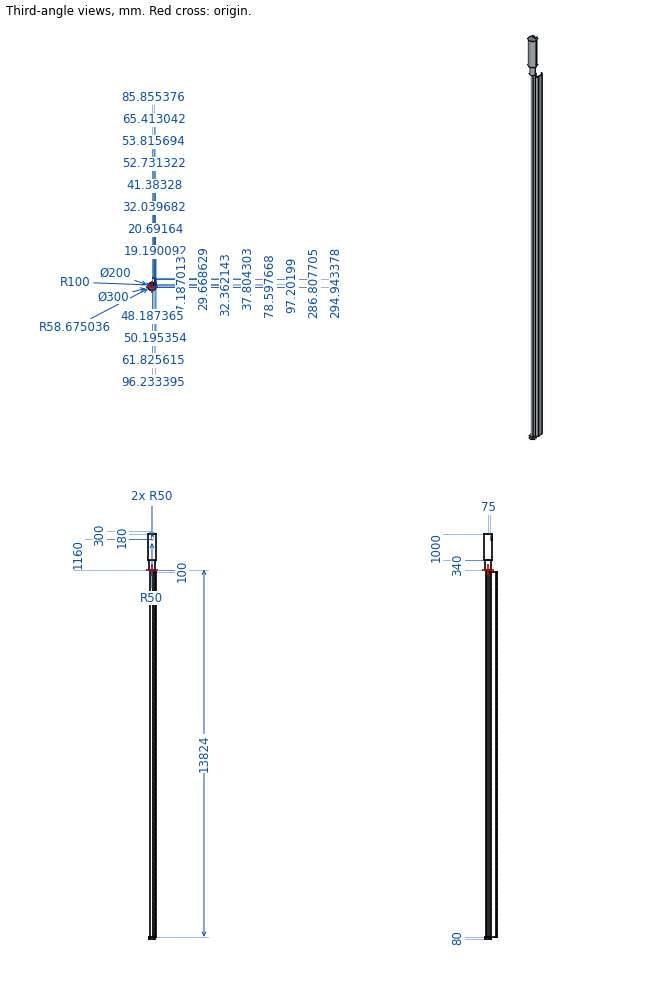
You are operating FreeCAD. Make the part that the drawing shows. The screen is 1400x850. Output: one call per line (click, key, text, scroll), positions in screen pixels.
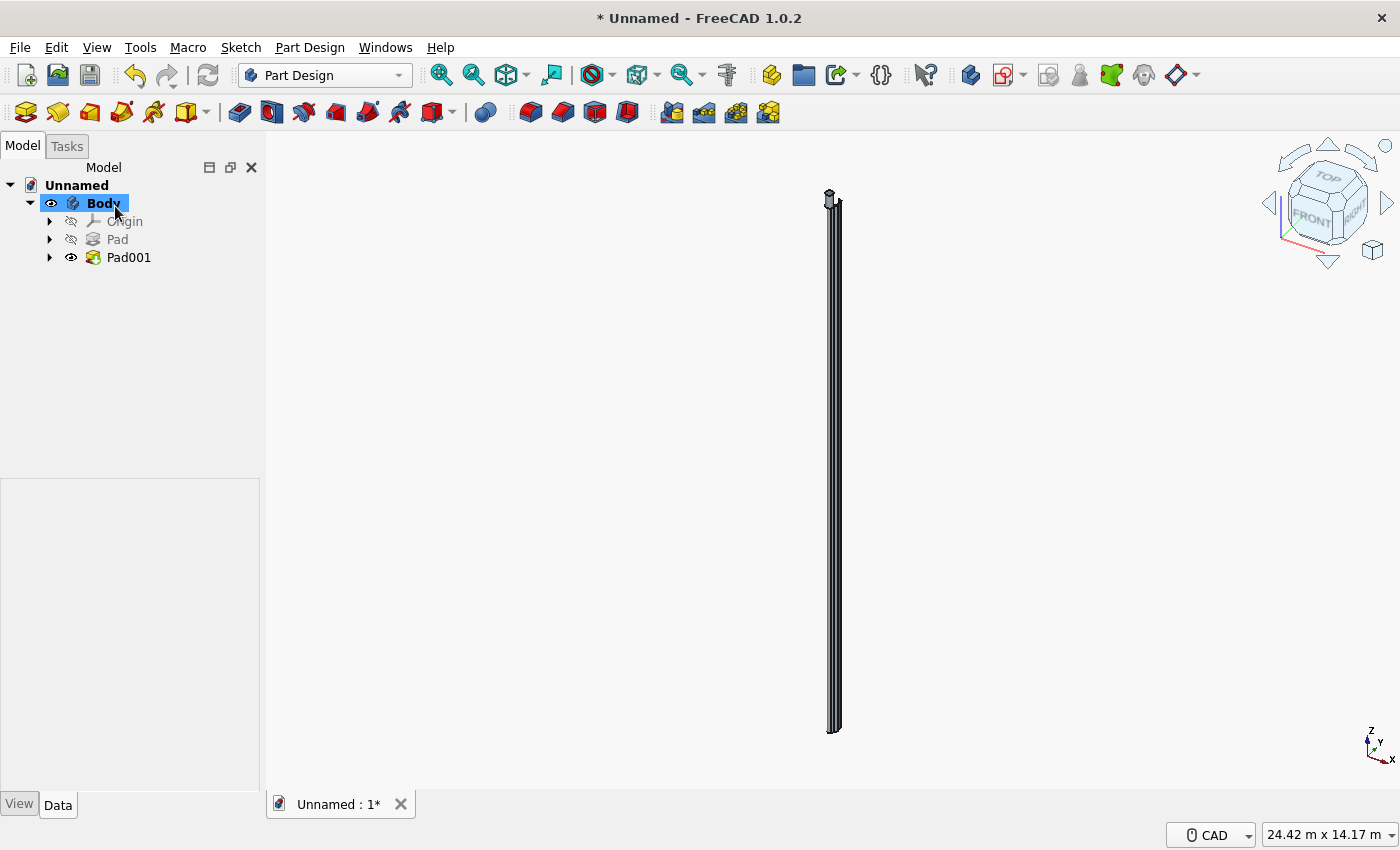
click(50, 221)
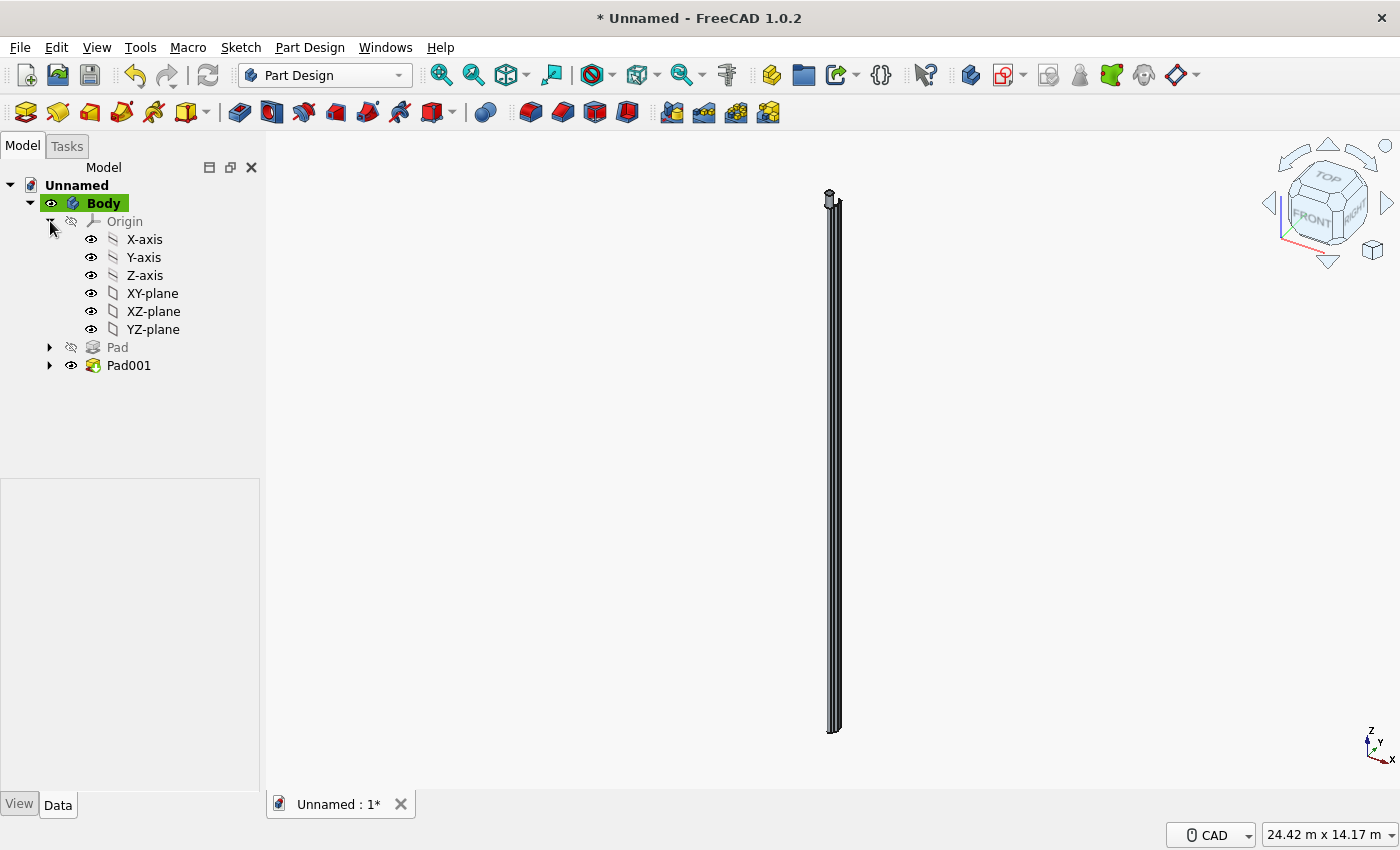
click(136, 293)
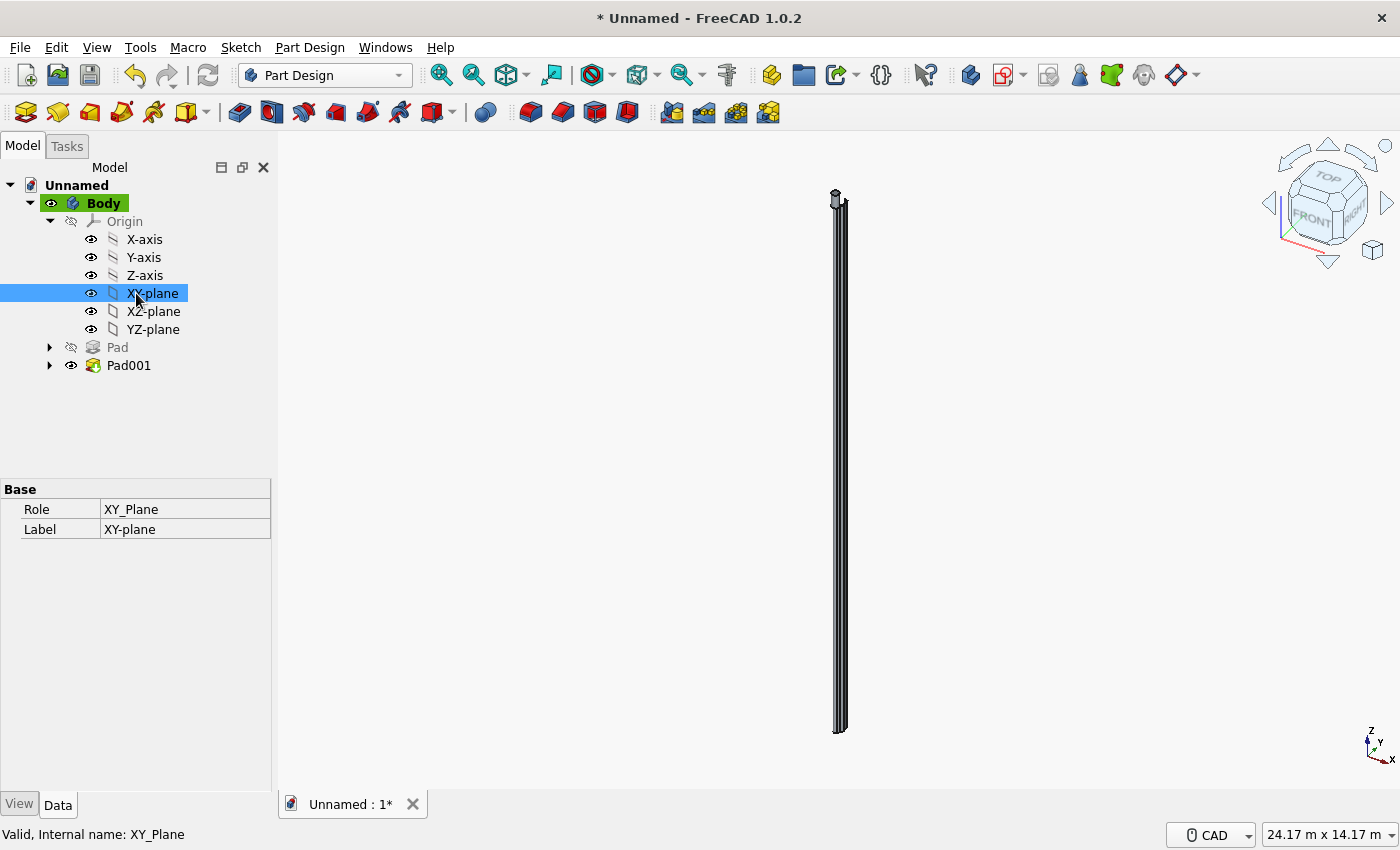
click(1176, 76)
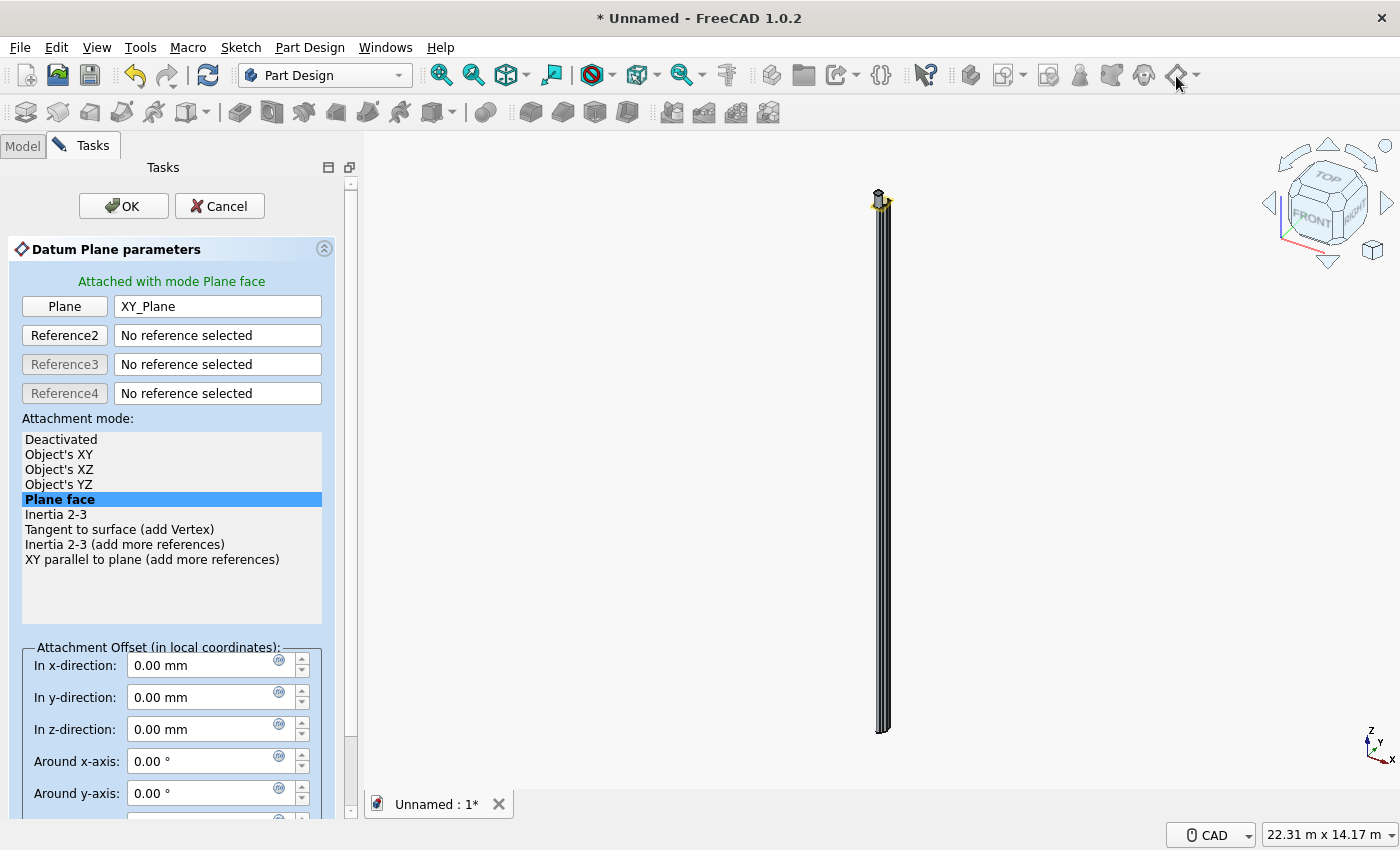
triple_click(210, 729)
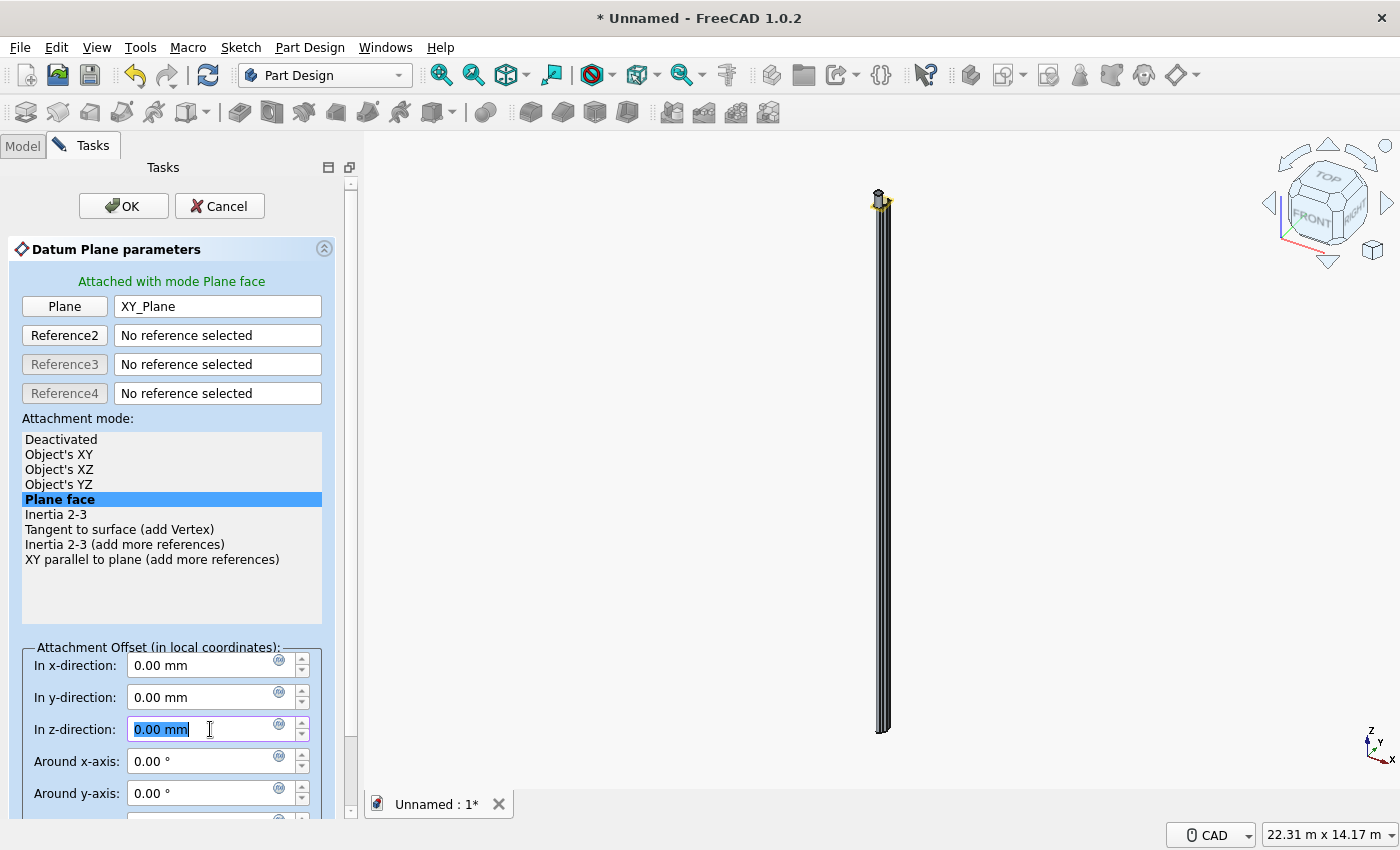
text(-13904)
key(Tab)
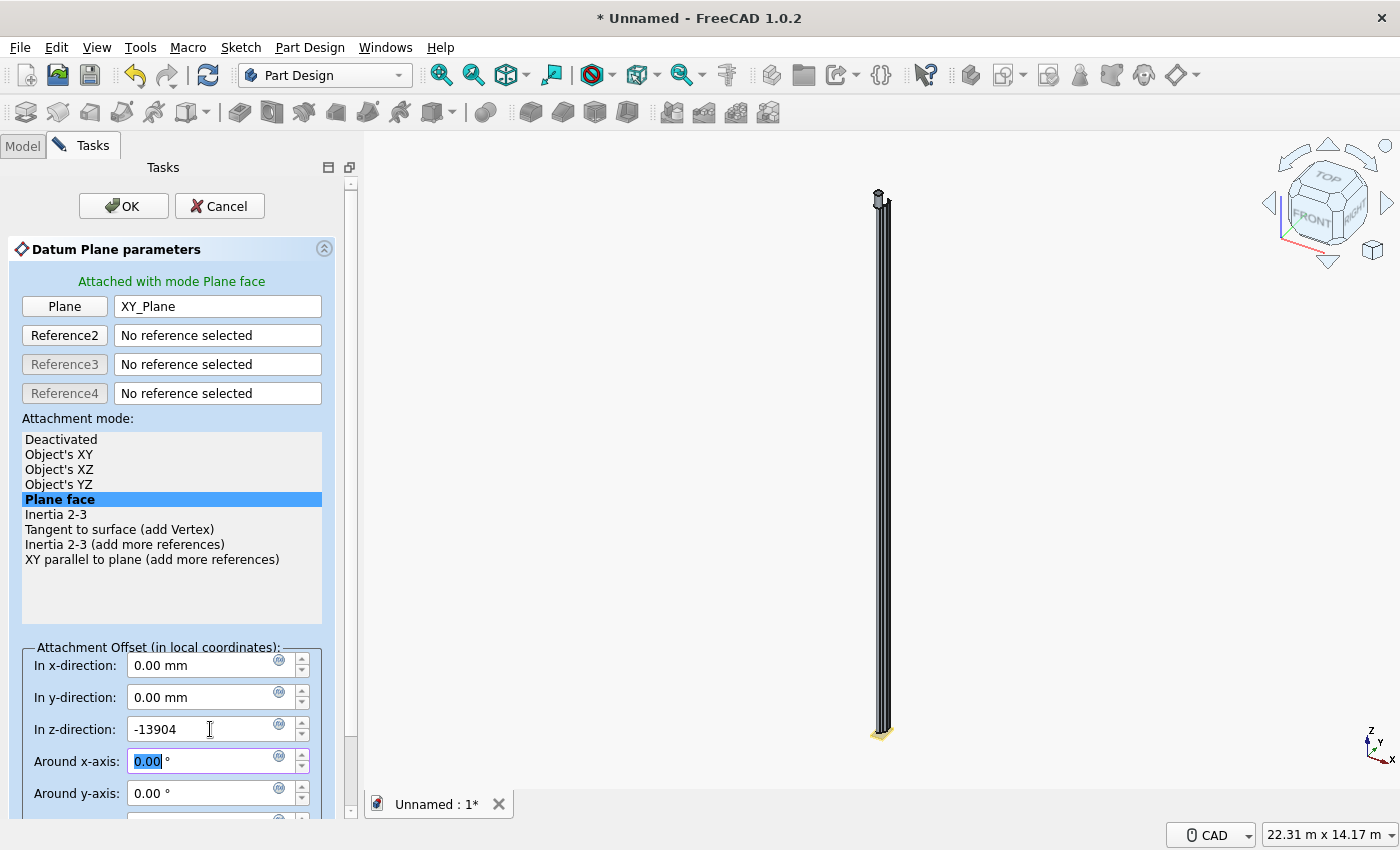
click(124, 206)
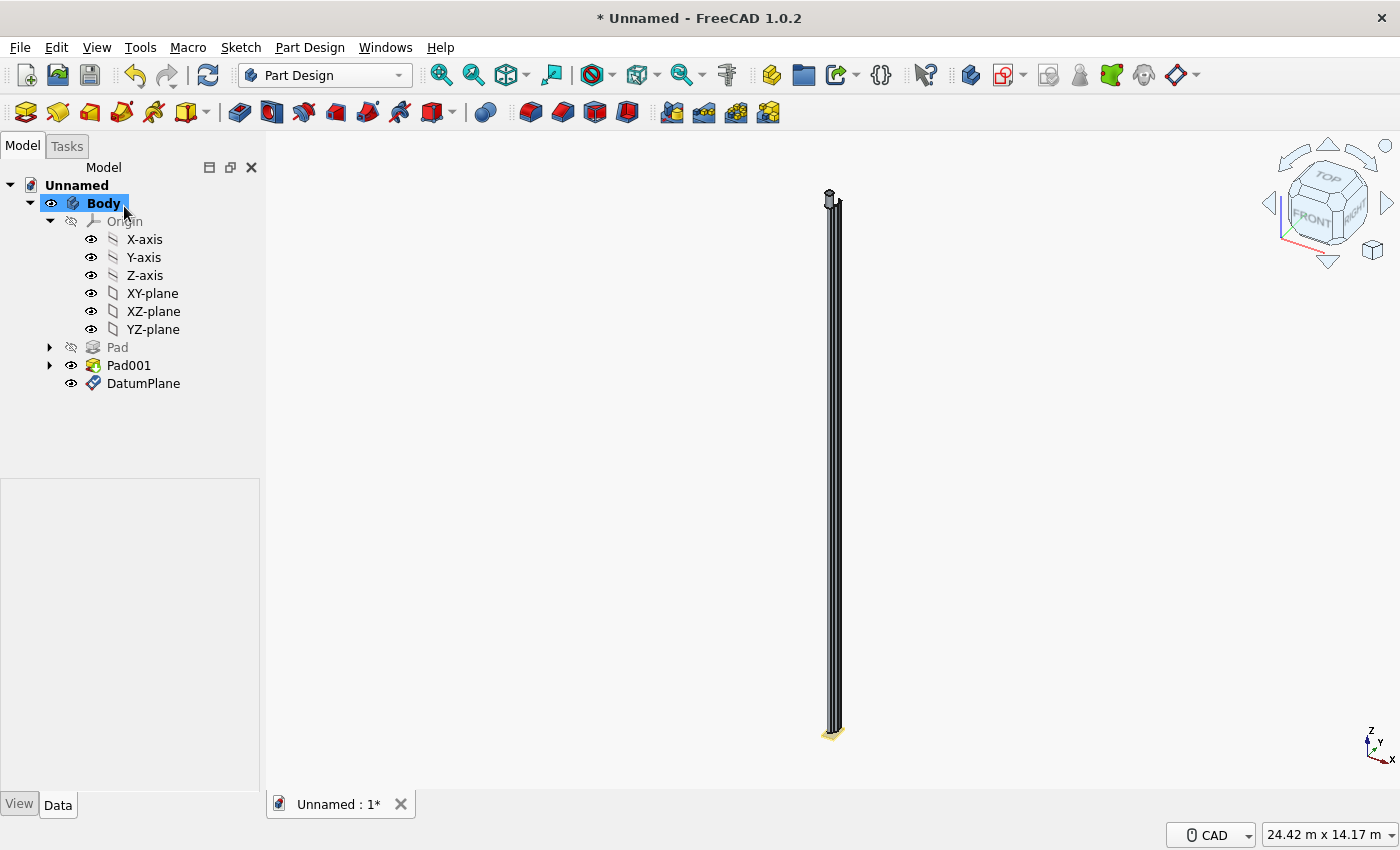
click(116, 383)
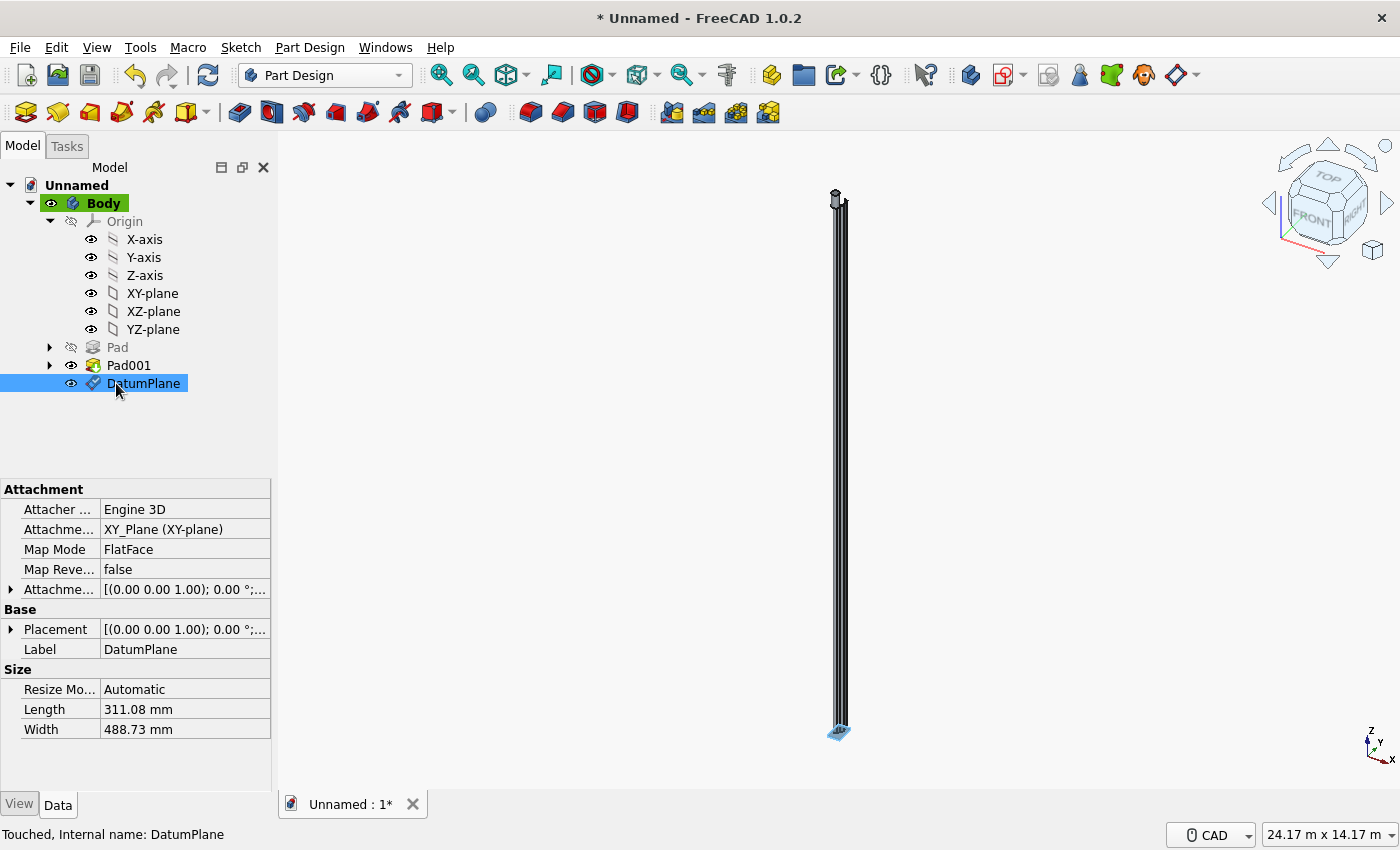
click(1004, 76)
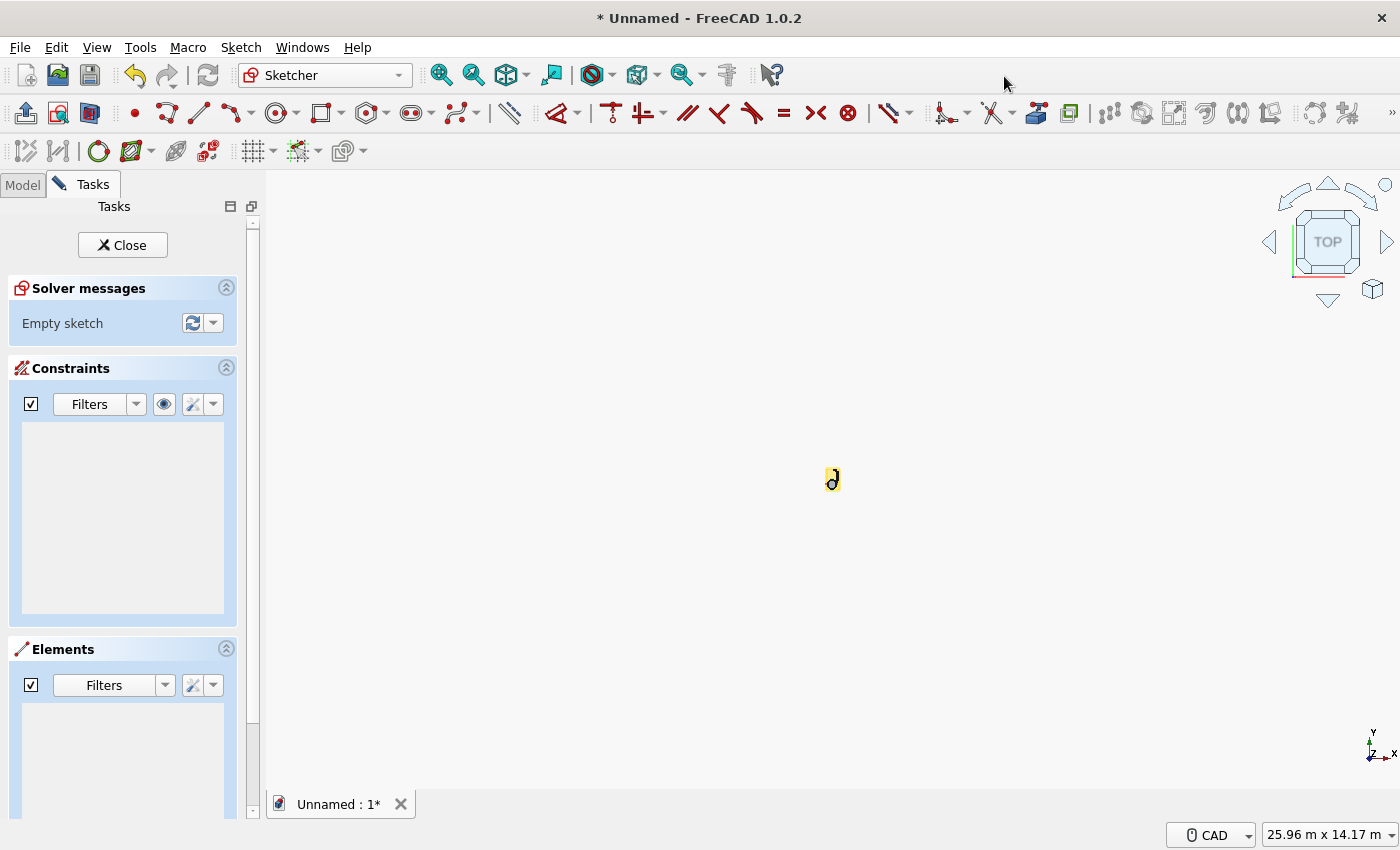
key(q)
key(s)